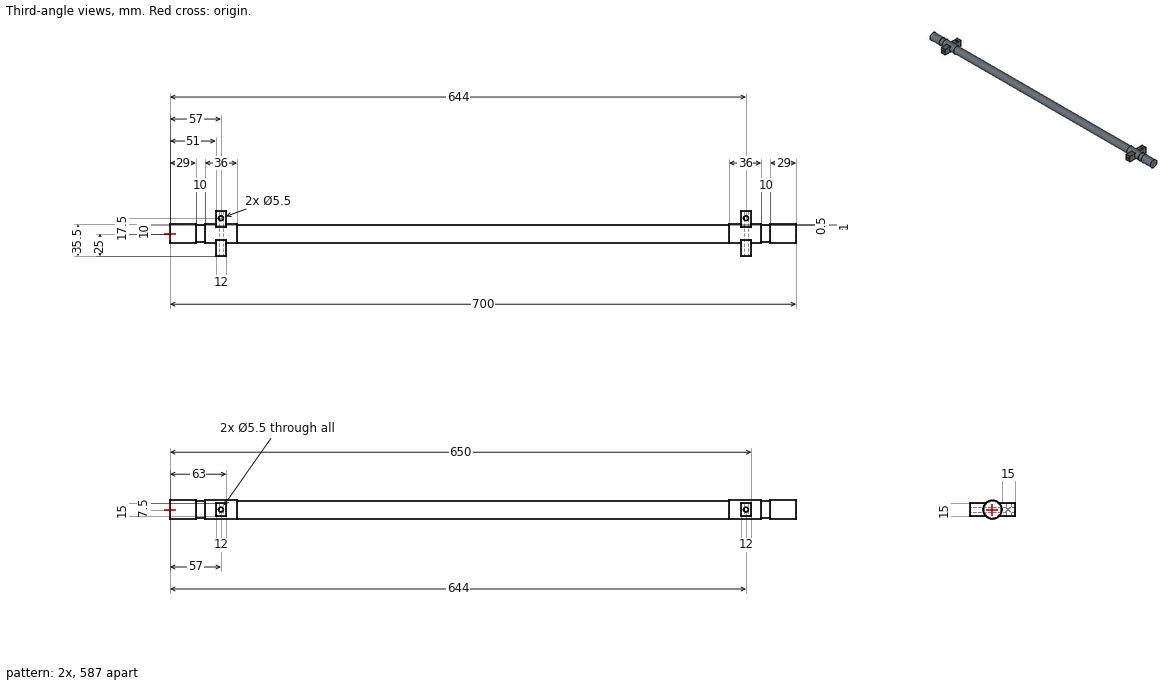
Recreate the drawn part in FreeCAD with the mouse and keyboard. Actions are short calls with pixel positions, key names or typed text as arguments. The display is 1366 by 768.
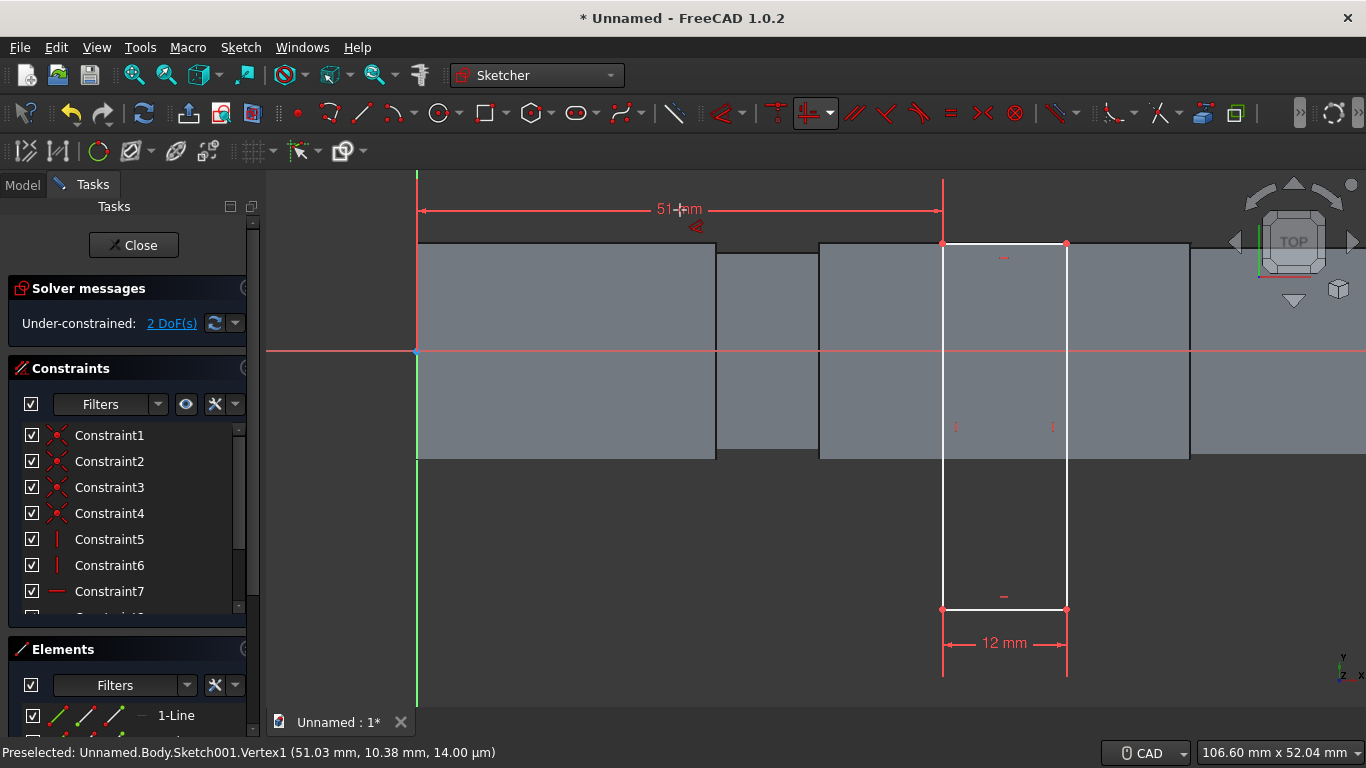
click(943, 610)
click(383, 481)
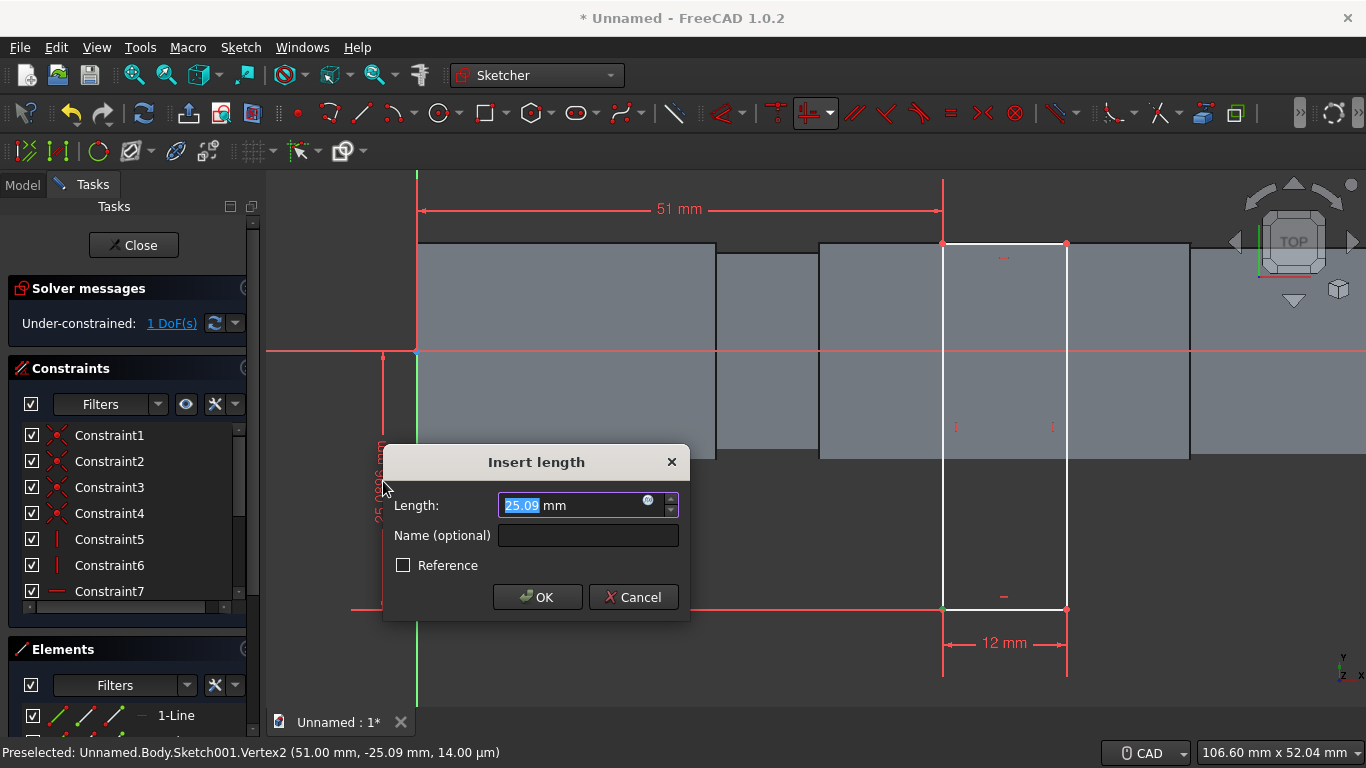
text(25)
key(Return)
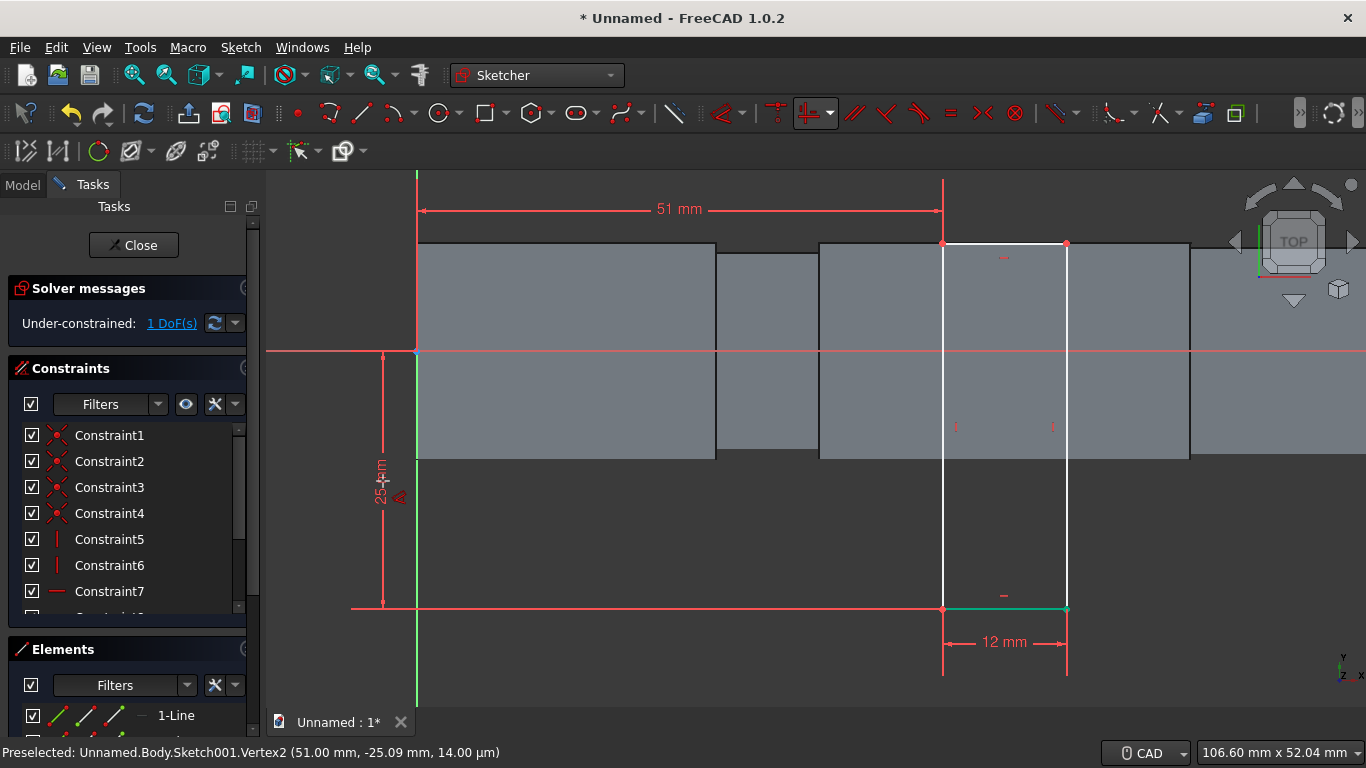
click(943, 354)
click(977, 427)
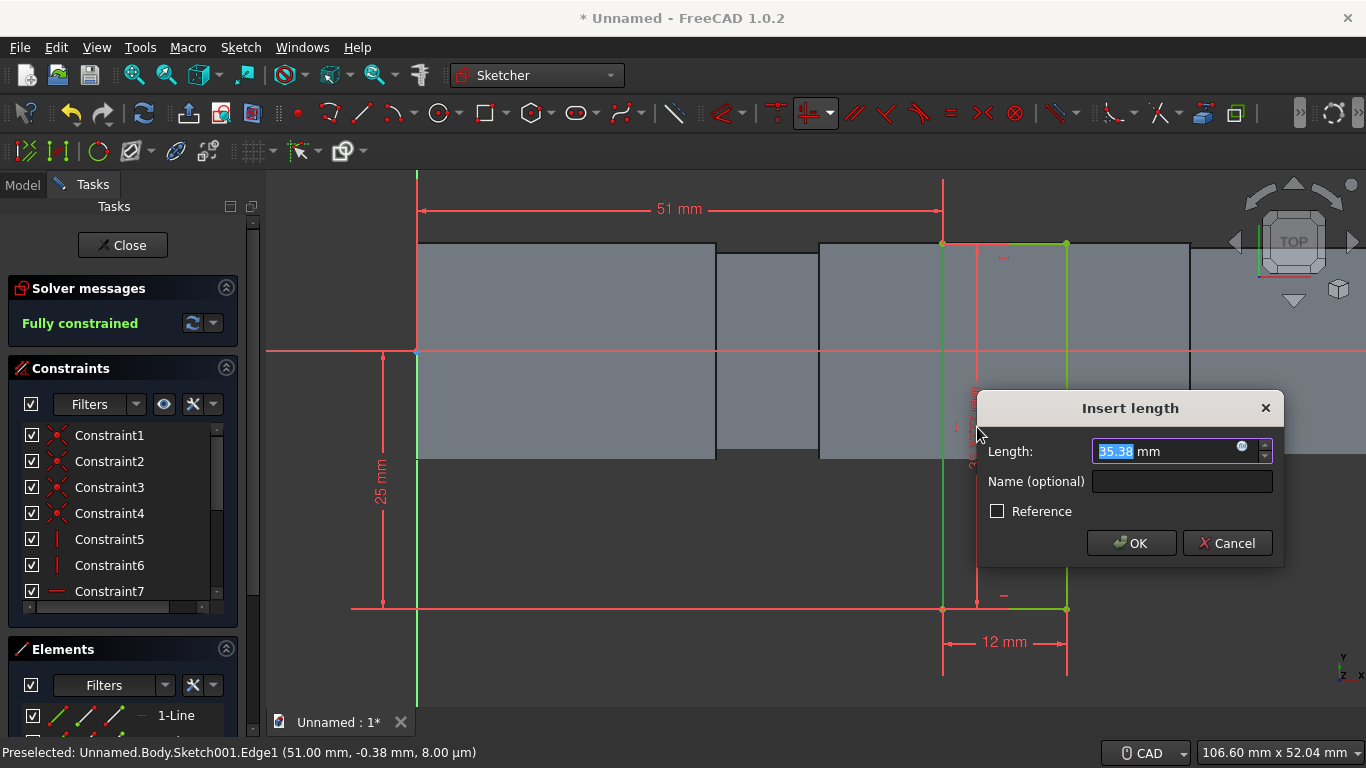
text(35.5)
key(Return)
key(Escape)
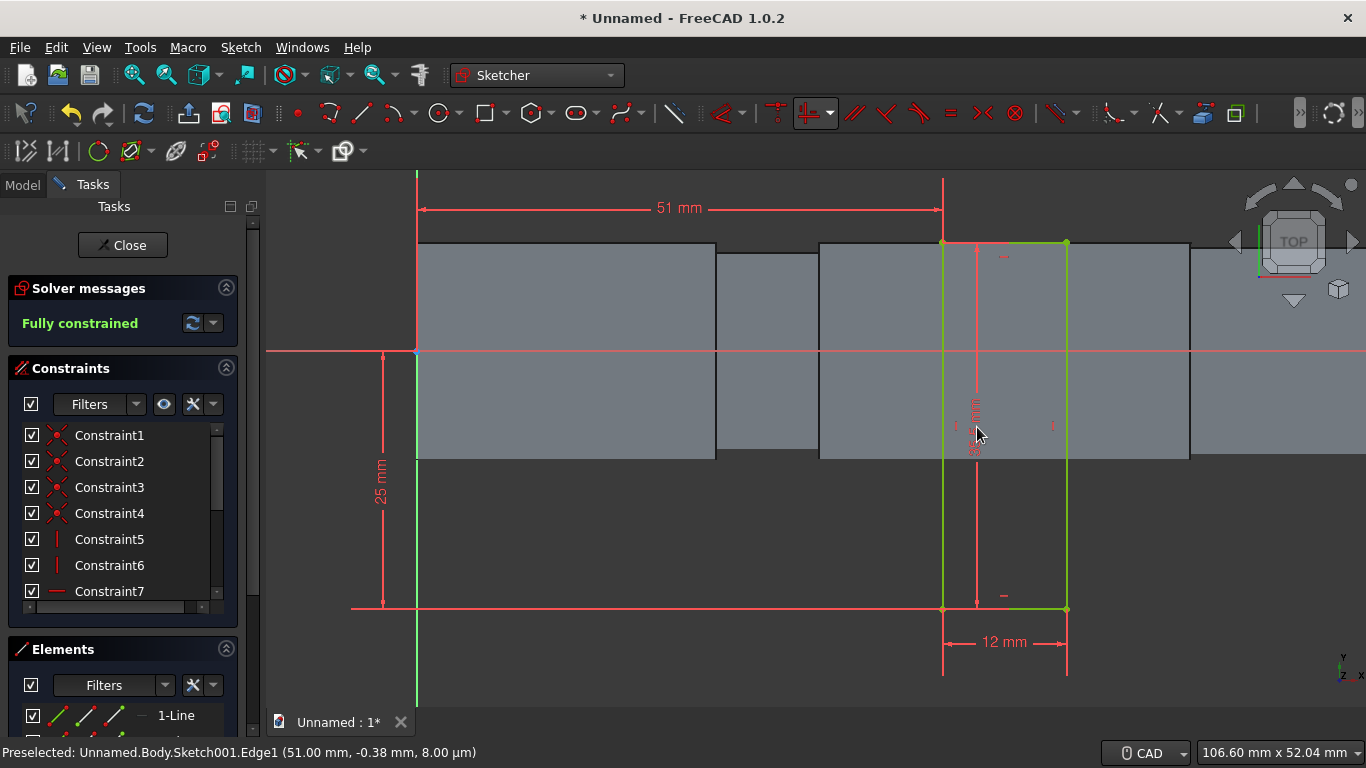
click(123, 245)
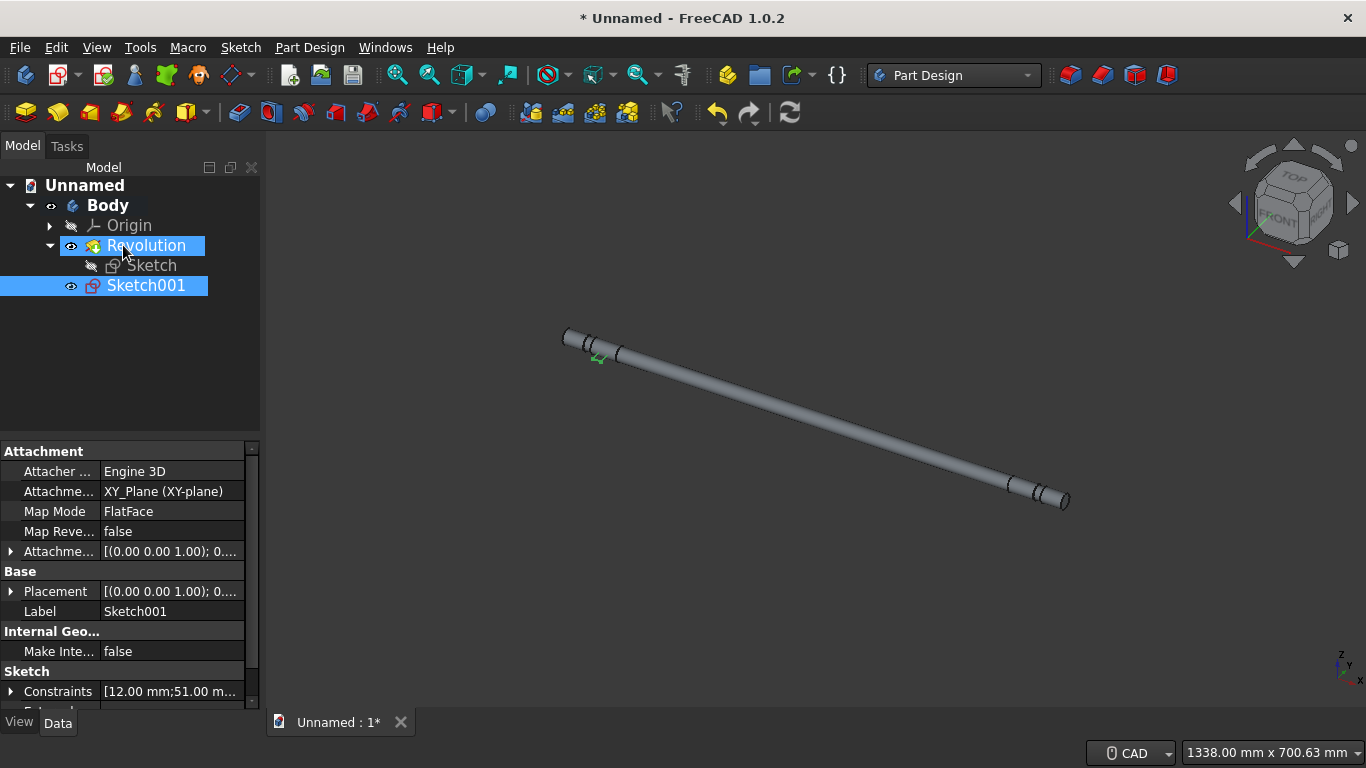
click(26, 112)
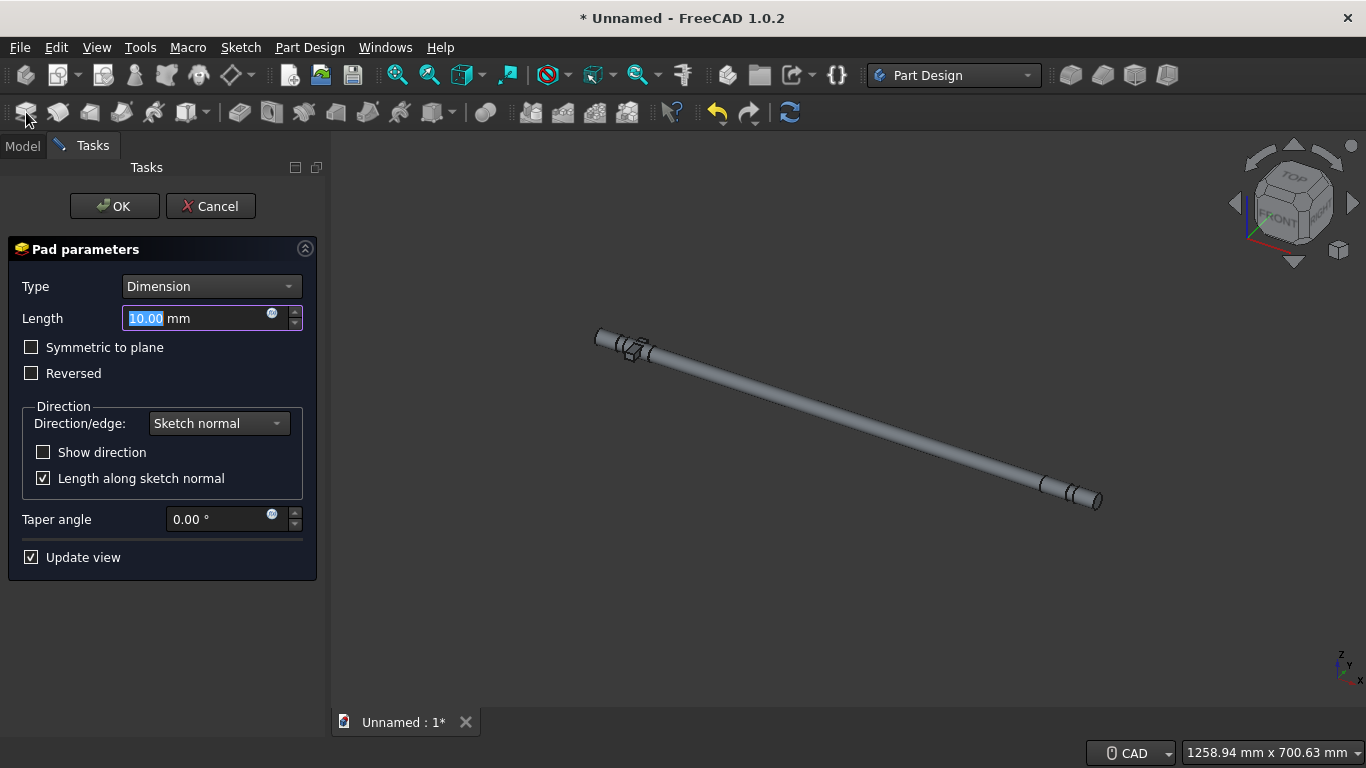
text(15)
key(Tab)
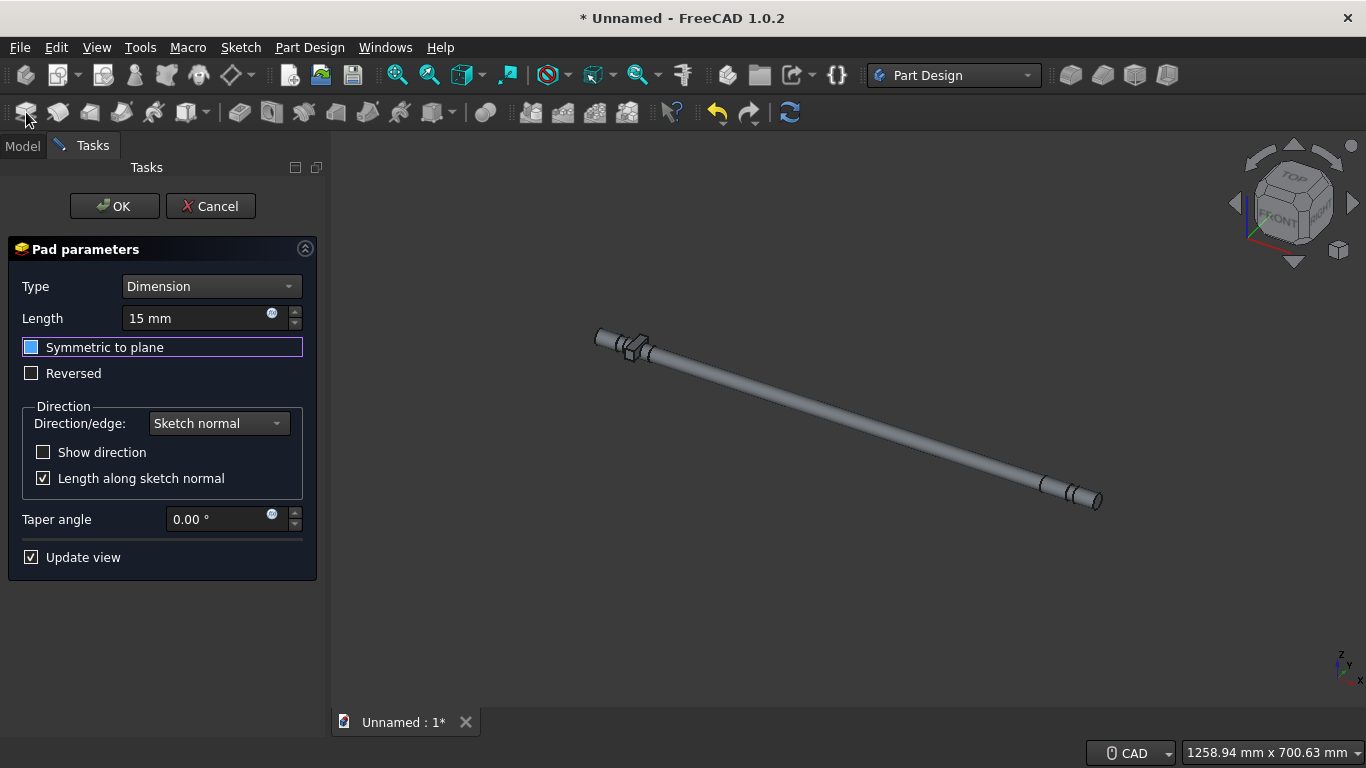
click(30, 347)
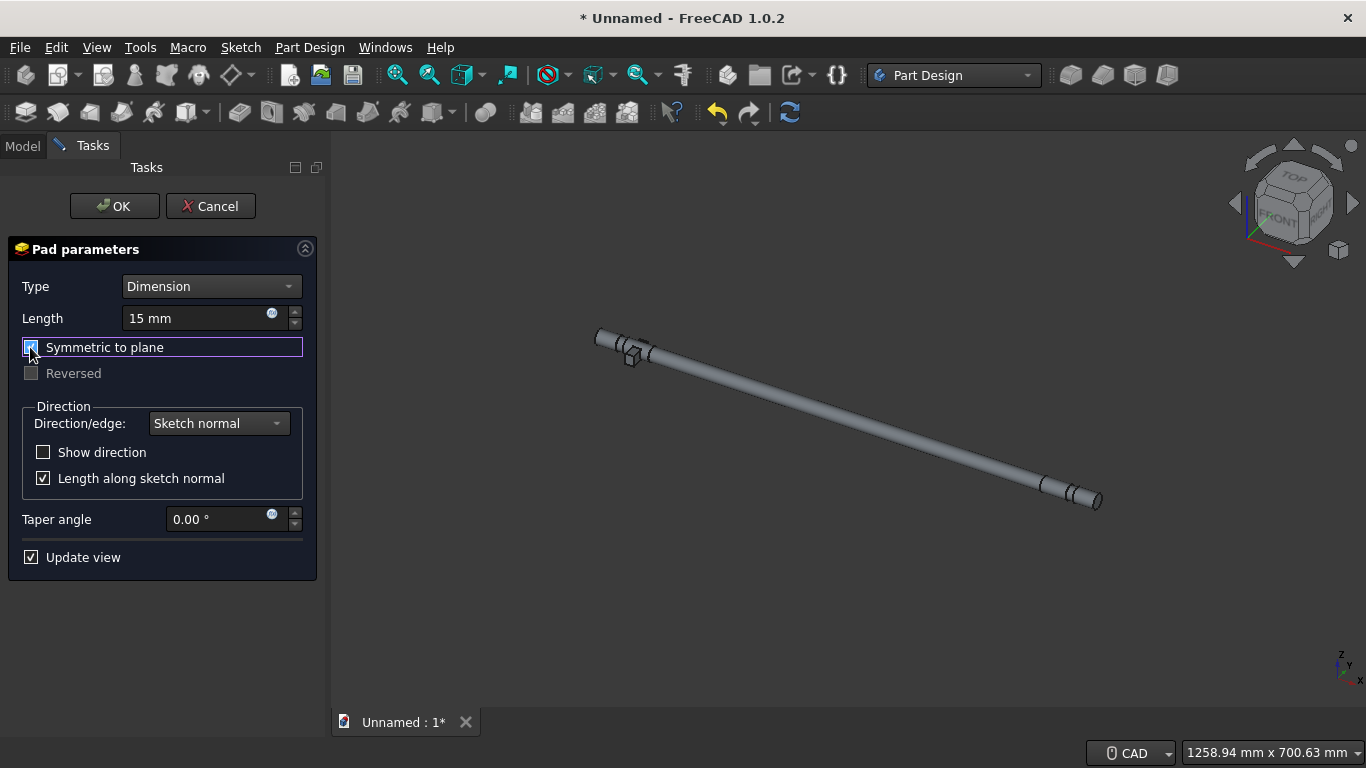
click(115, 206)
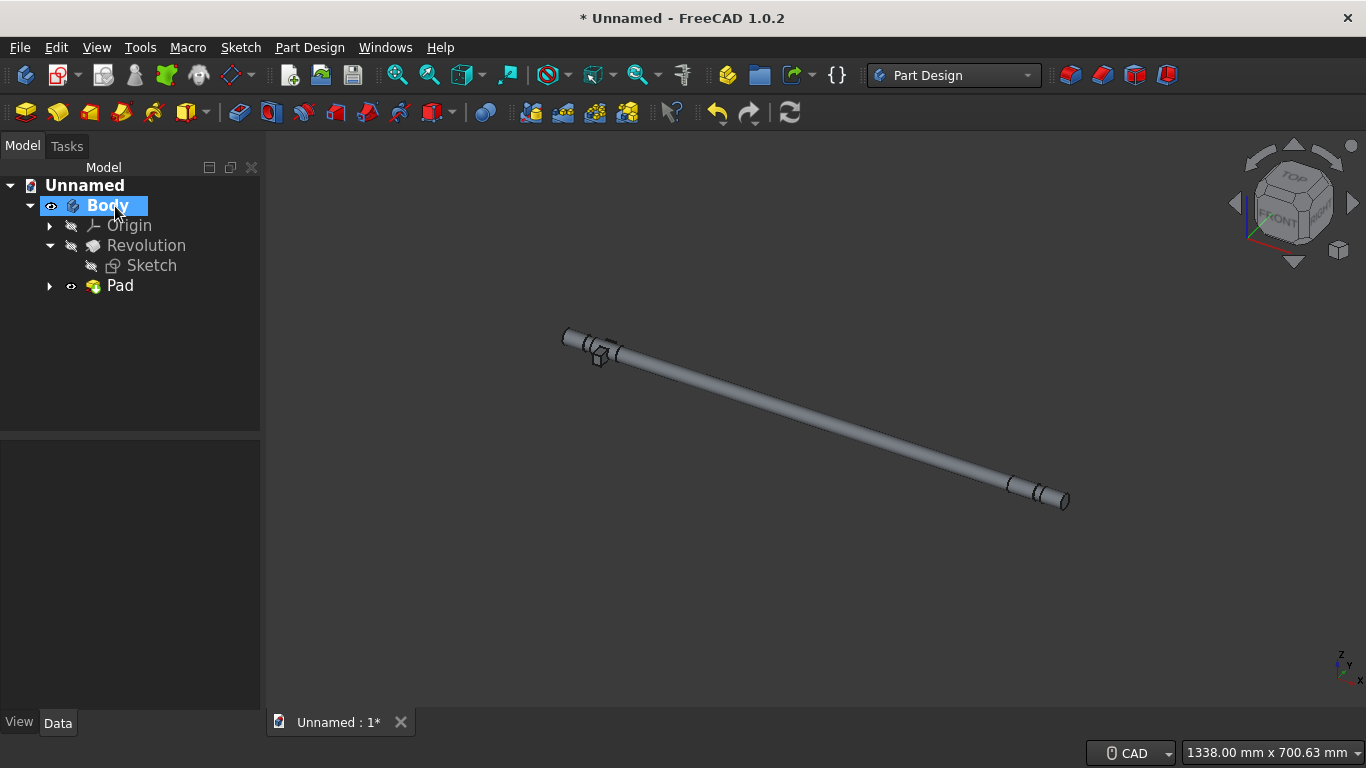
click(116, 286)